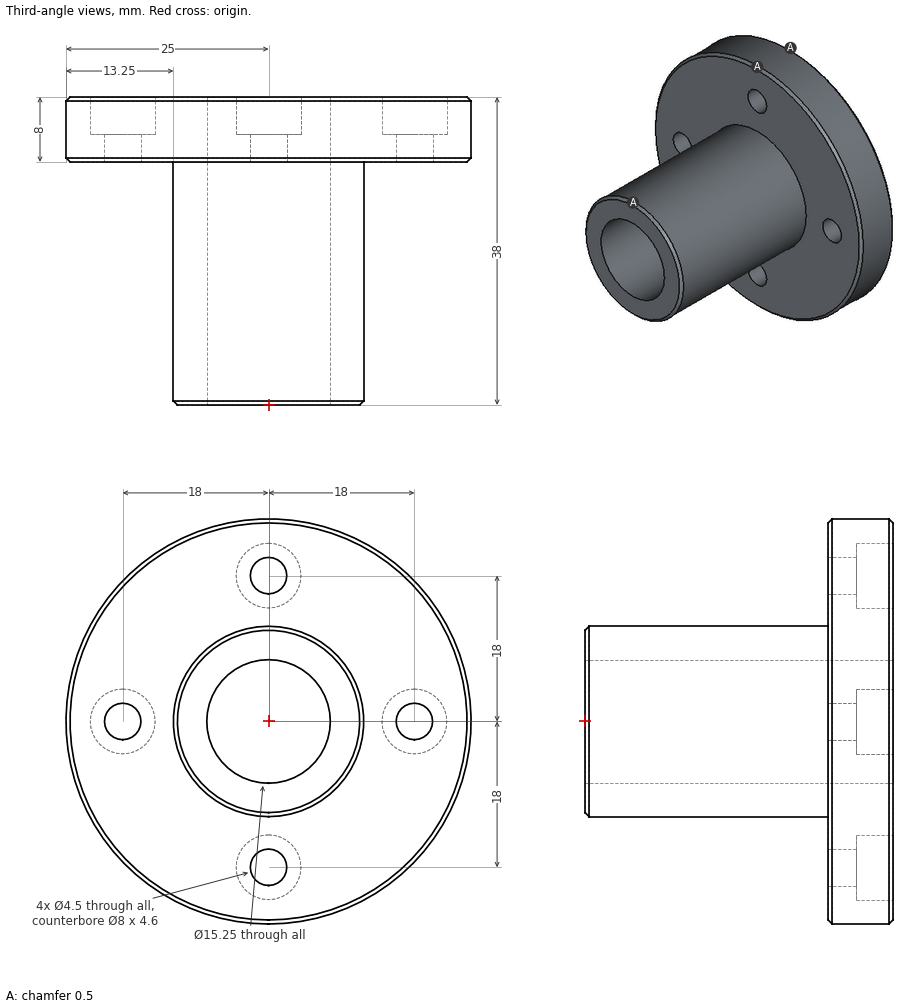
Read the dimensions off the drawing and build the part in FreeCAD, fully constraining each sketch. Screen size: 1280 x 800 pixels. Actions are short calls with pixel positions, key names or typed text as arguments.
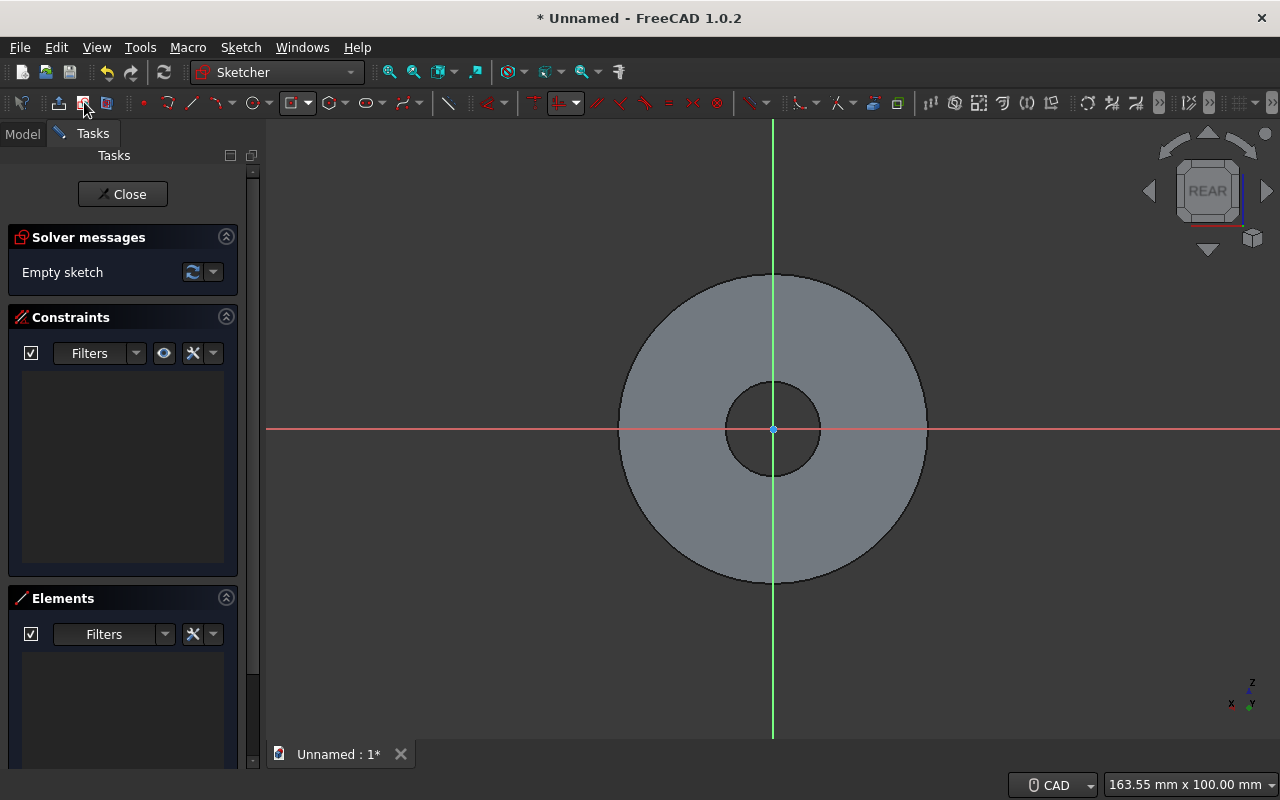
scroll(912, 429, up, 2)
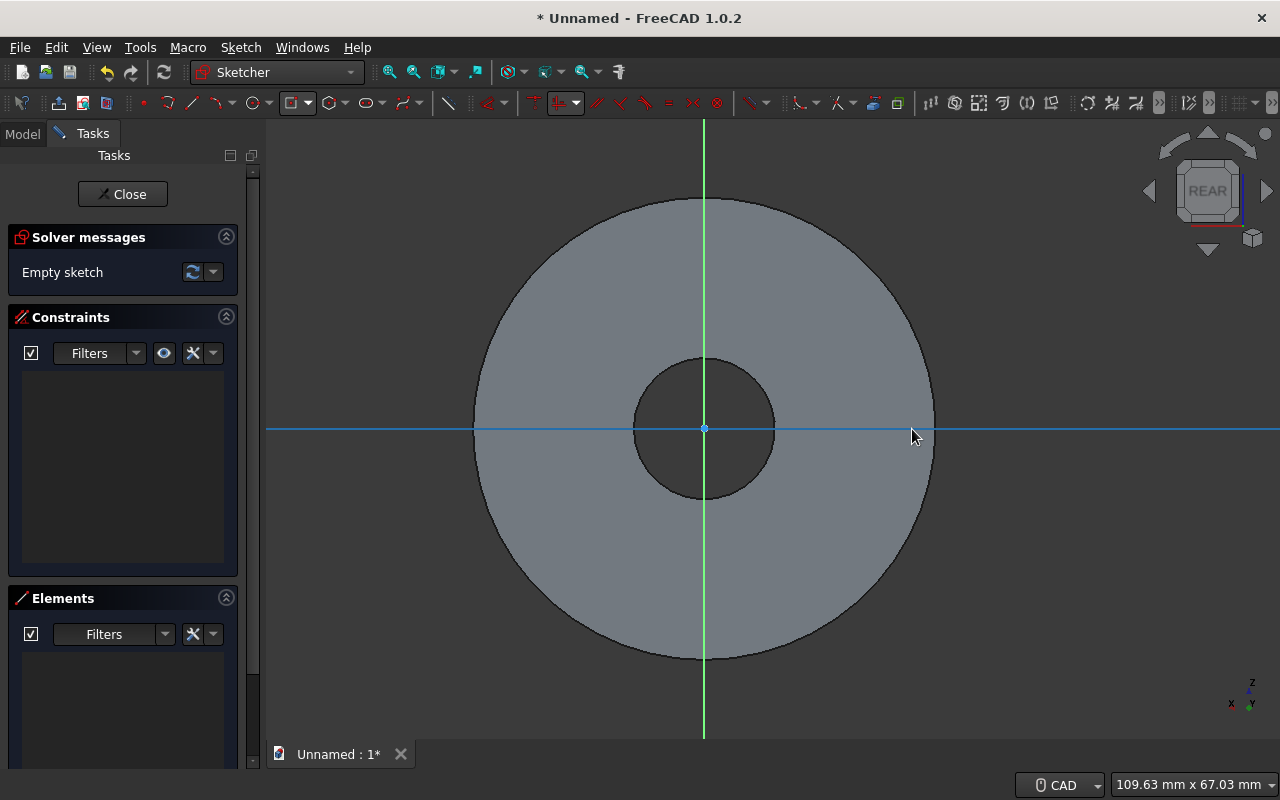
click(254, 104)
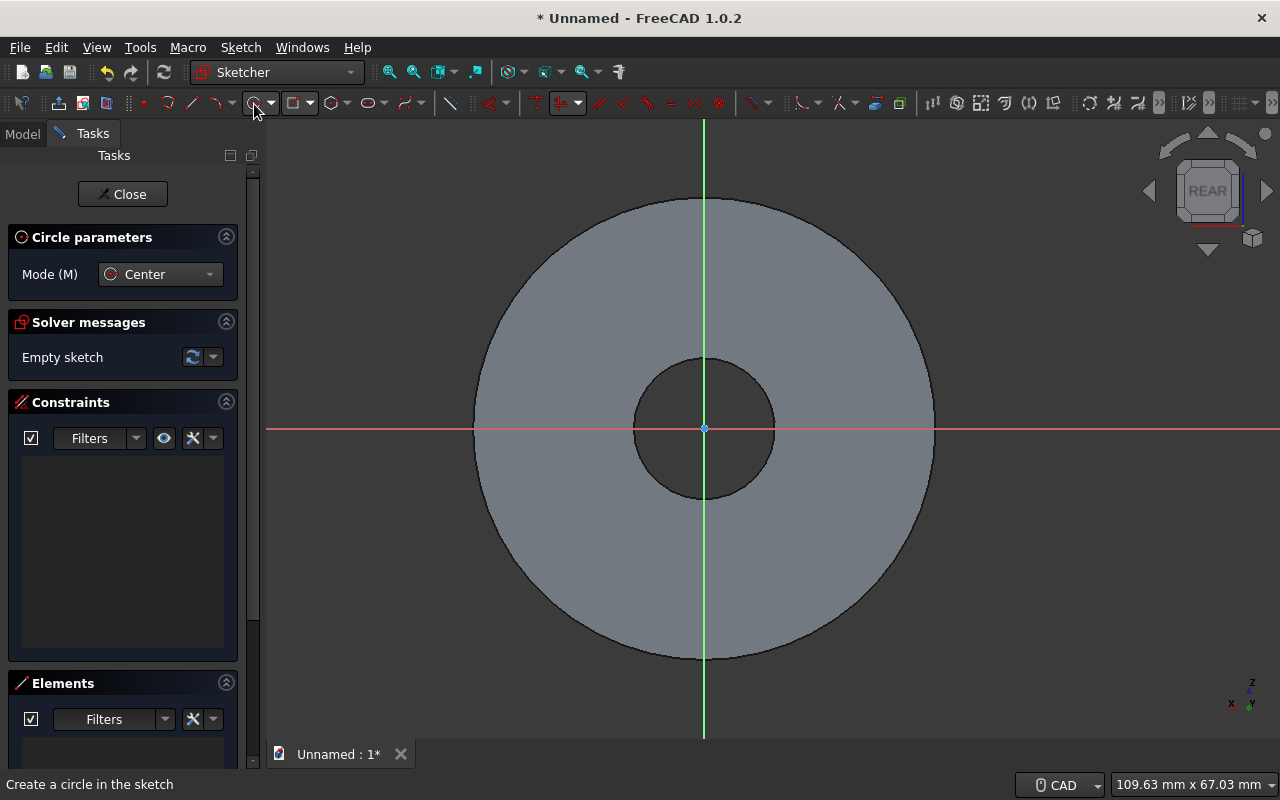
click(704, 595)
click(719, 581)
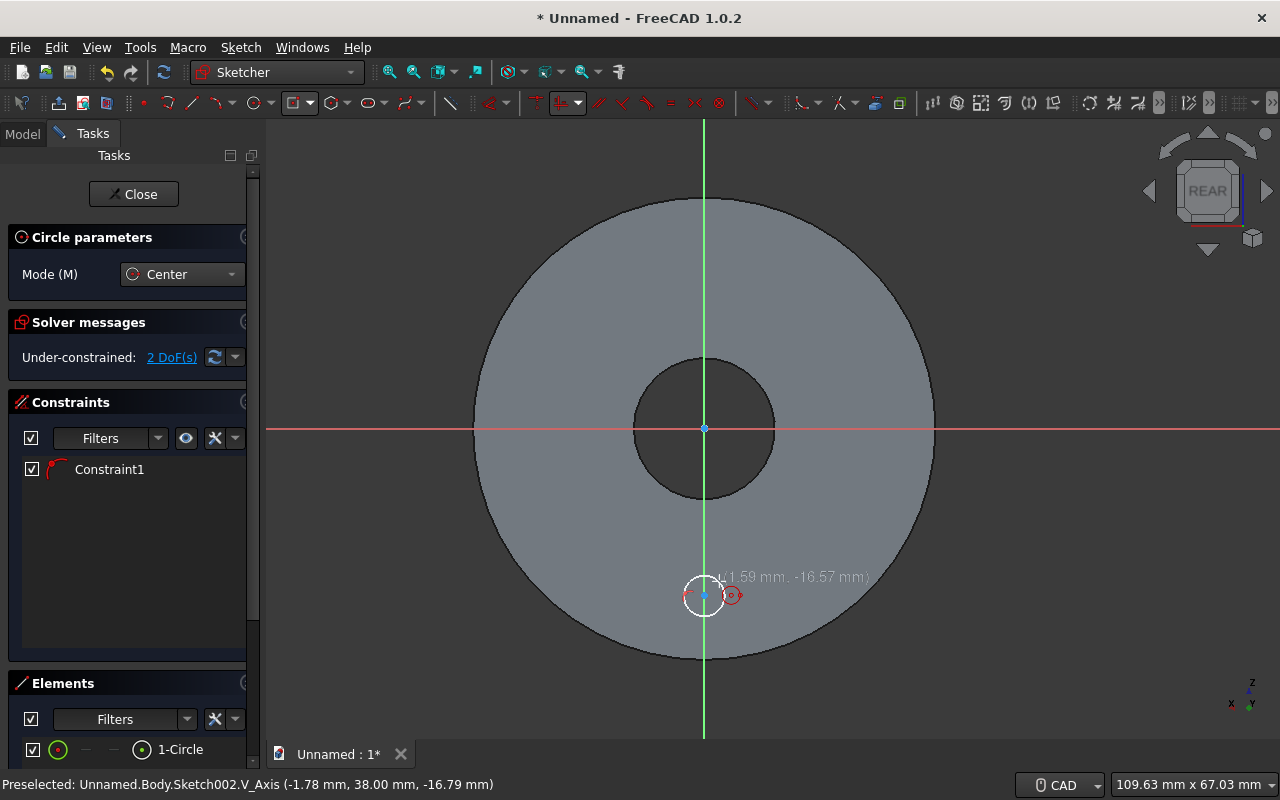
click(871, 429)
click(886, 414)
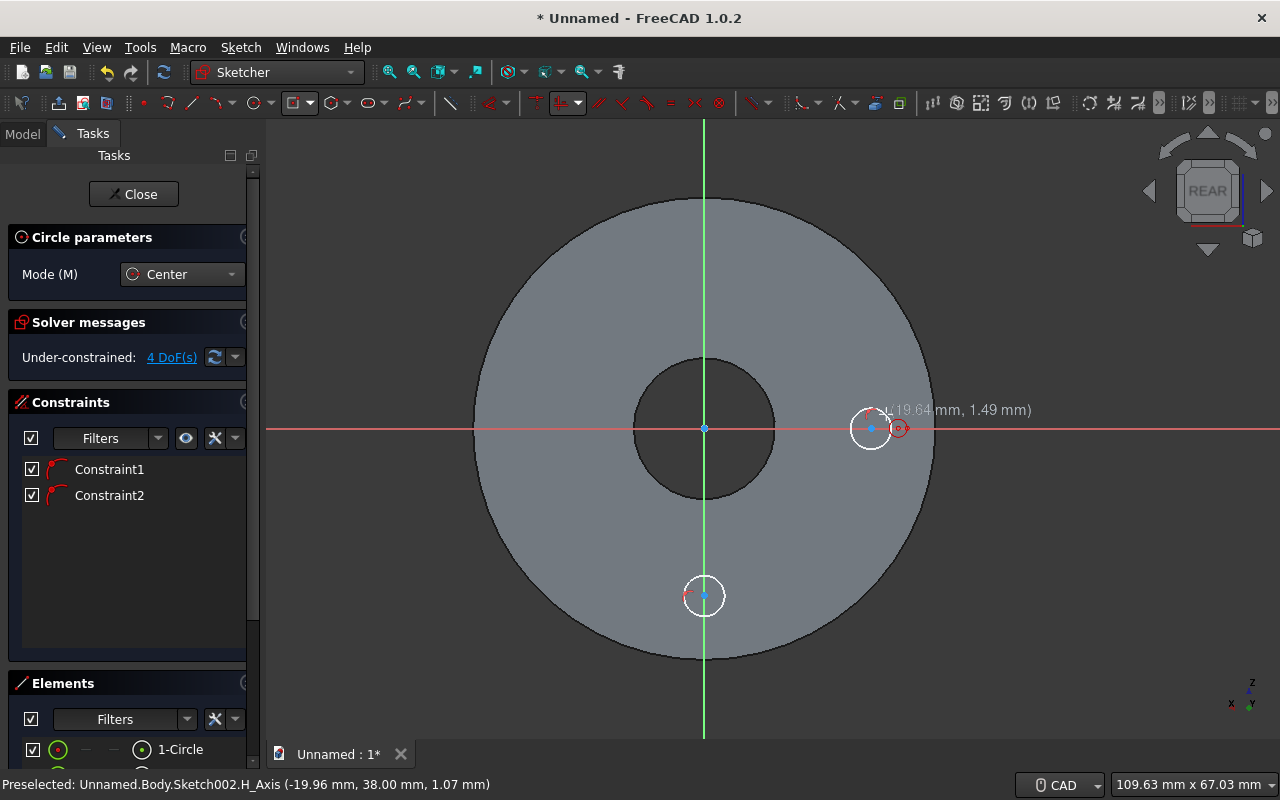
click(538, 429)
click(553, 414)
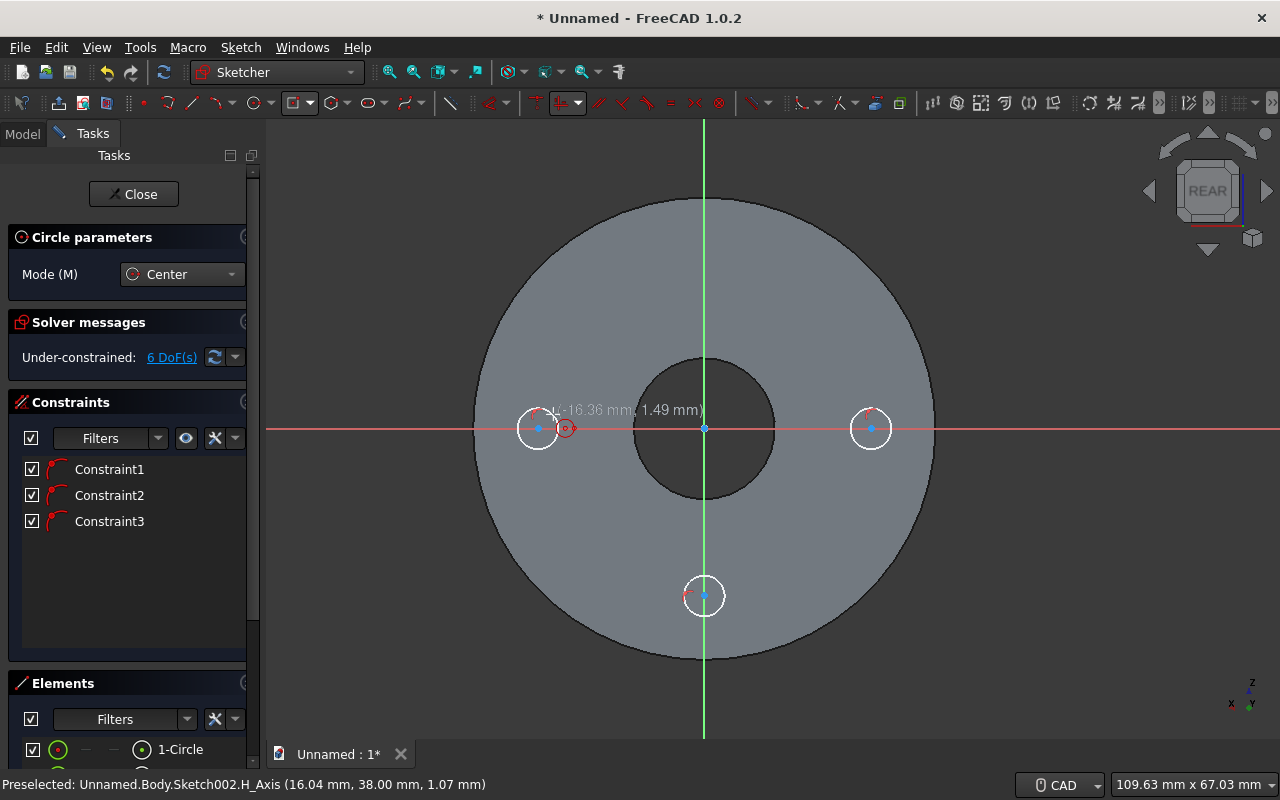
click(704, 262)
click(719, 248)
key(Escape)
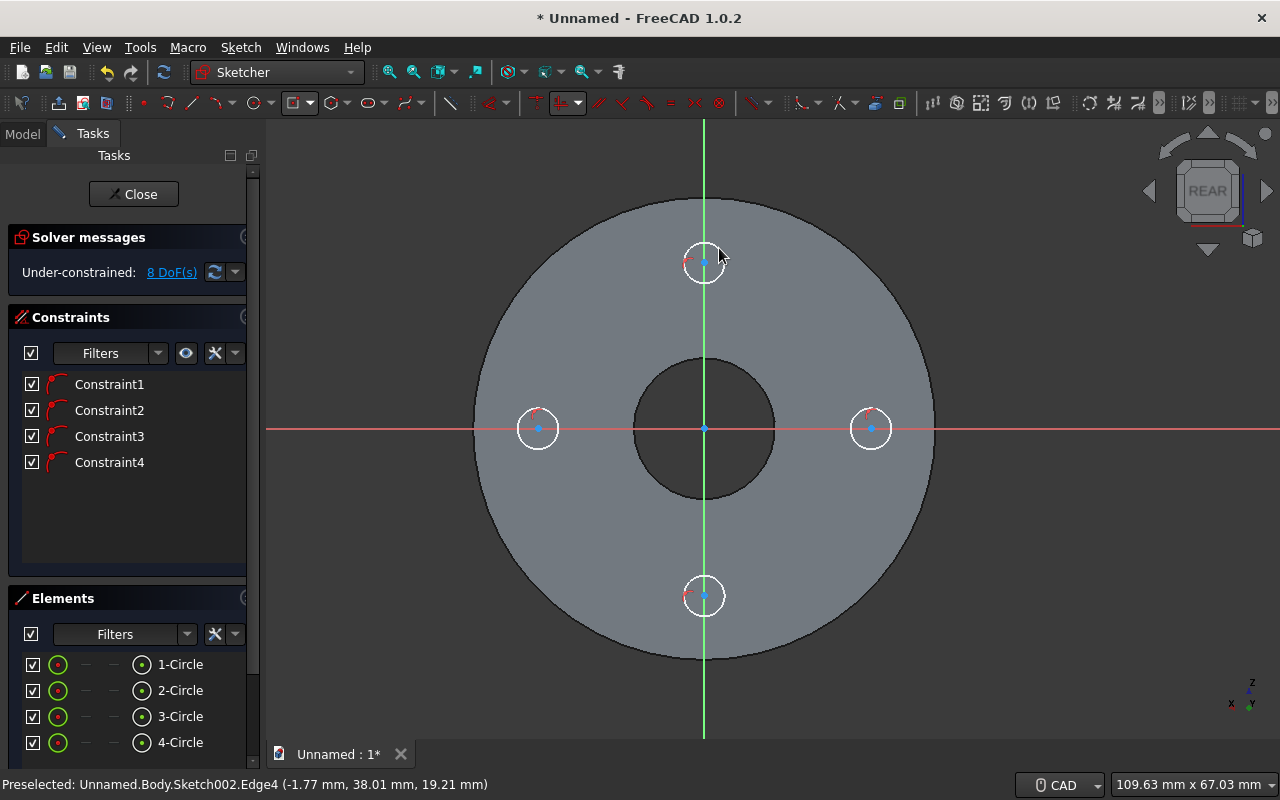
click(719, 582)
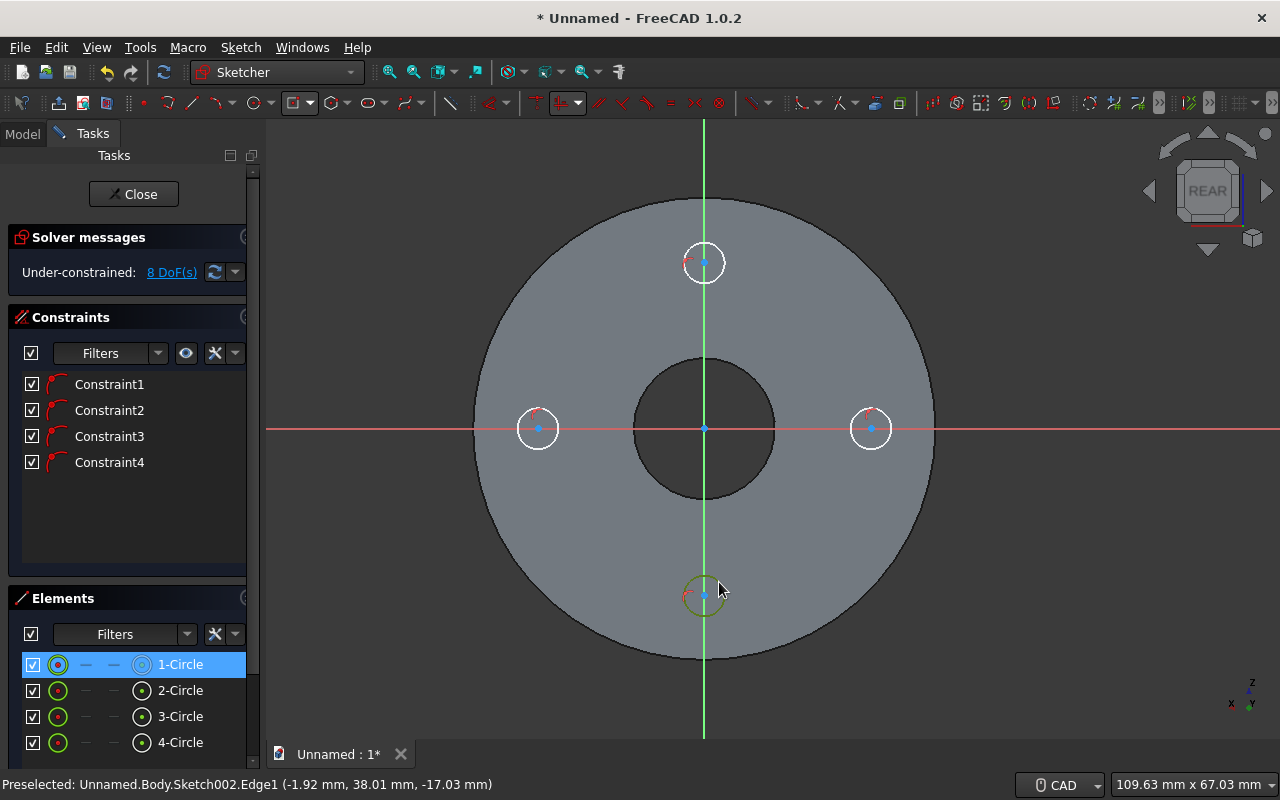
click(885, 414)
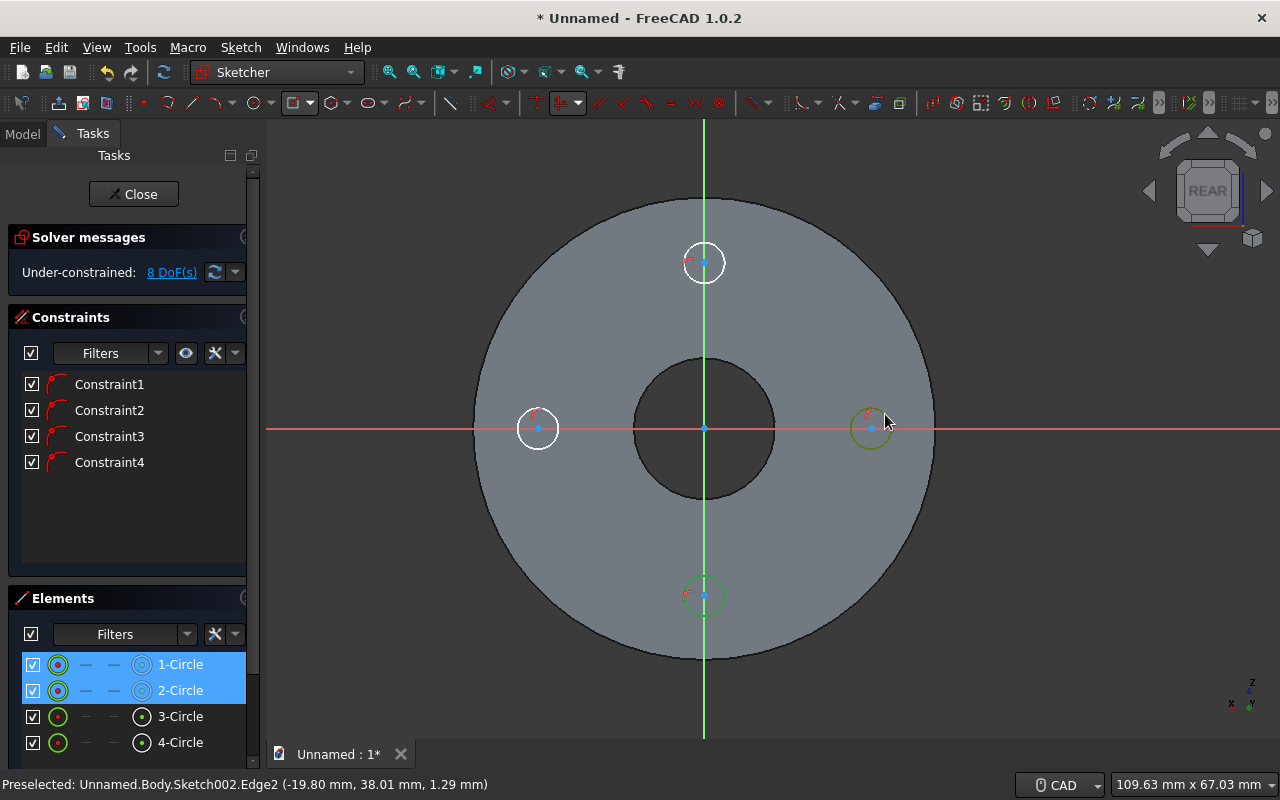
click(552, 414)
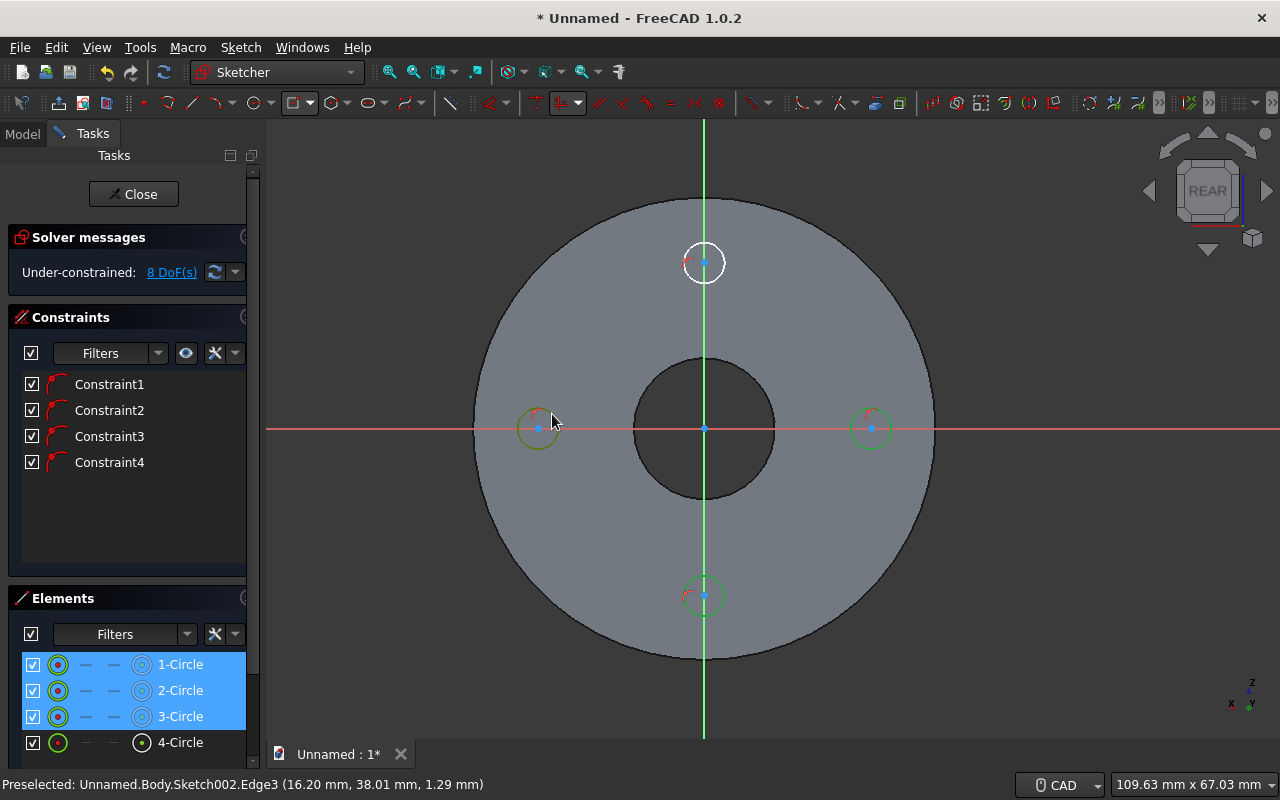
click(719, 249)